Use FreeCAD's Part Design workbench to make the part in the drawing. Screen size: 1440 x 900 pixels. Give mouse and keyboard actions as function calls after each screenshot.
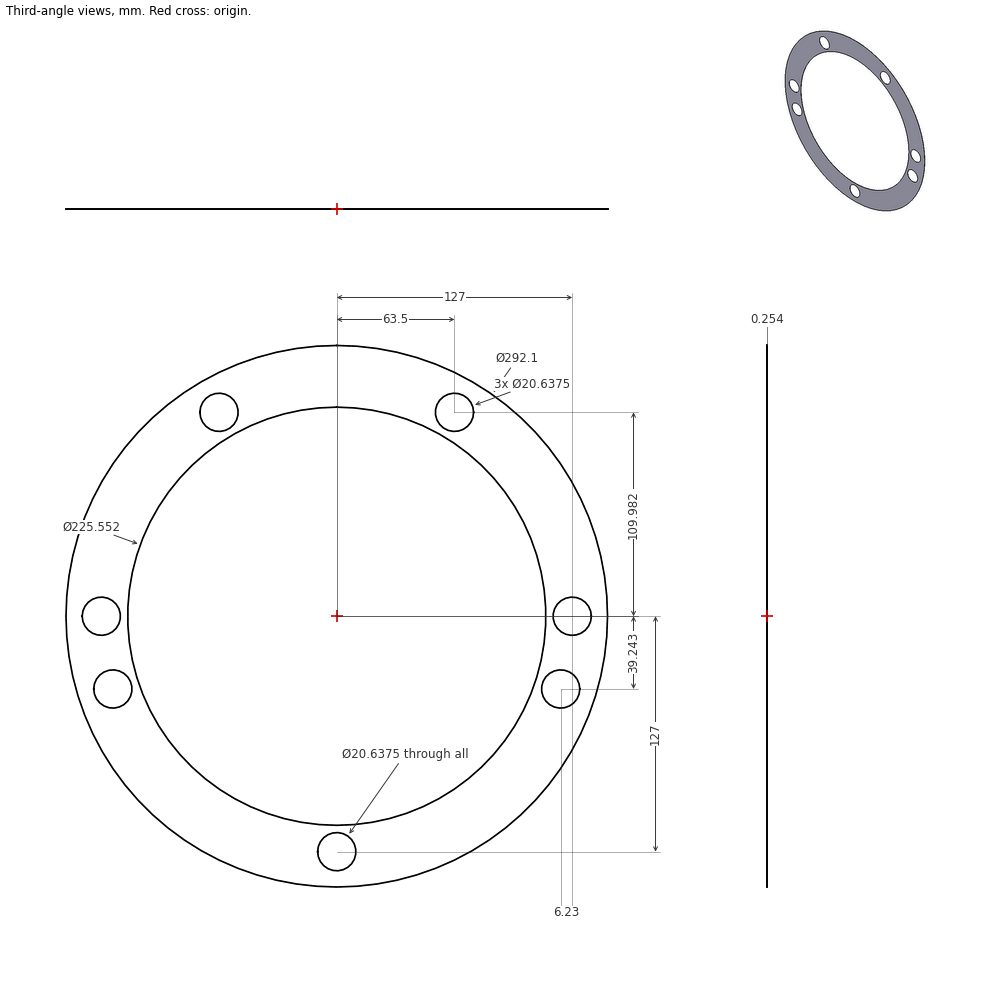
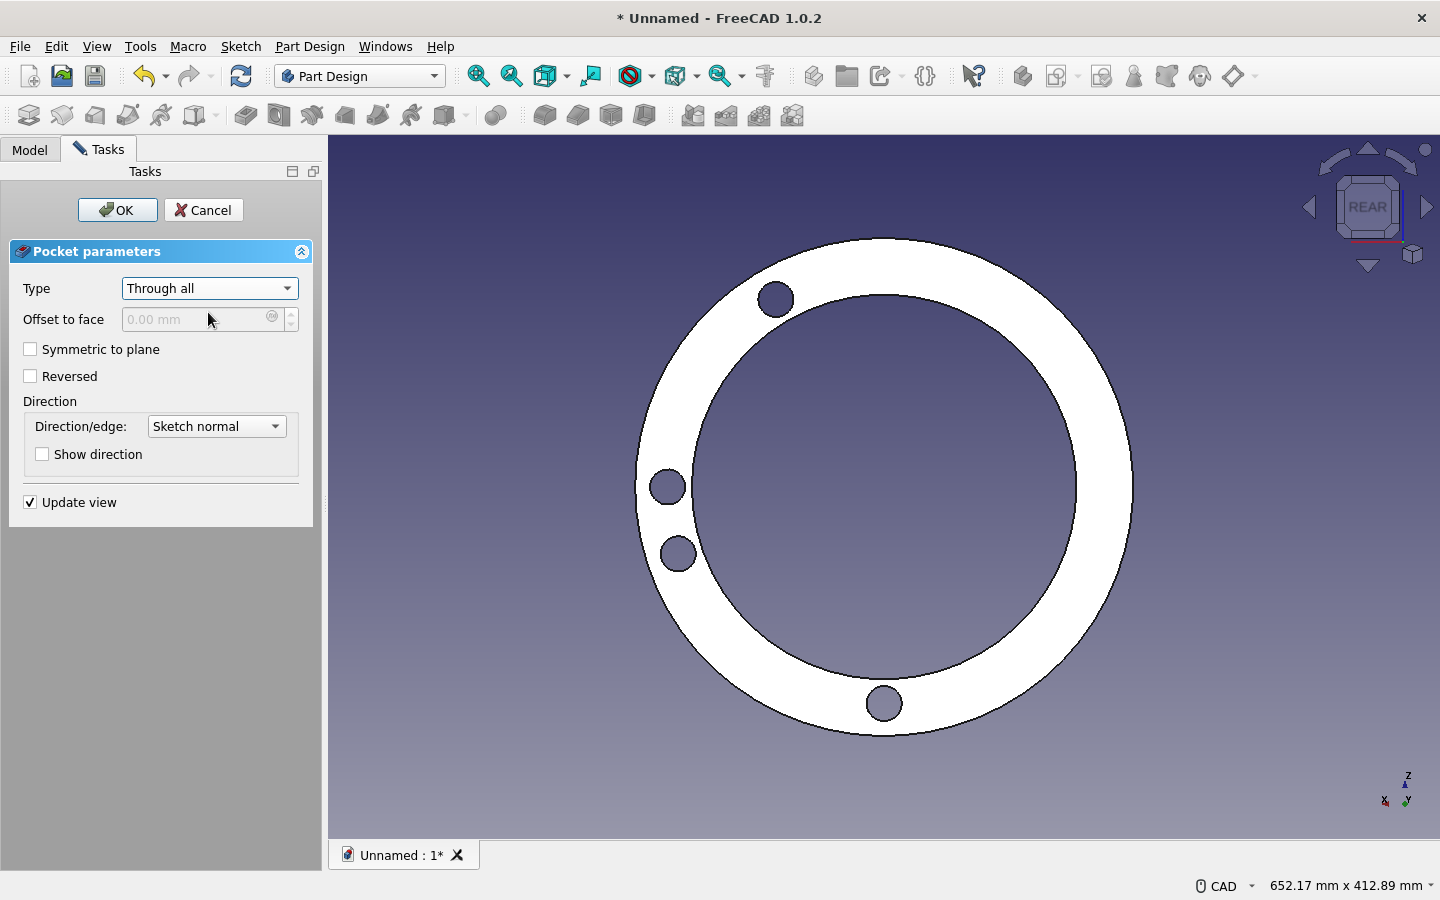
click(118, 210)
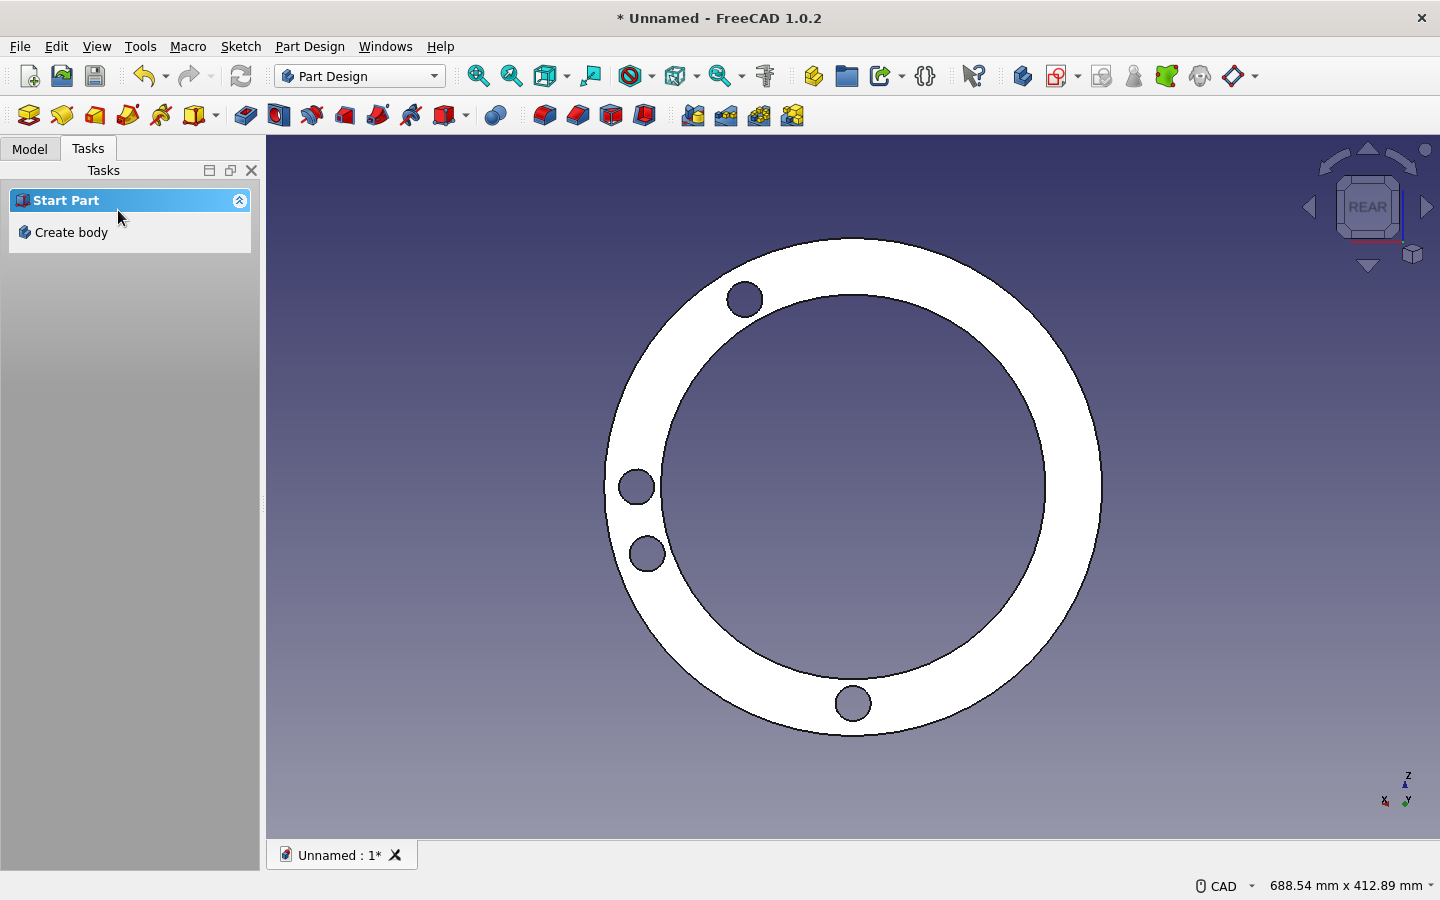
click(30, 148)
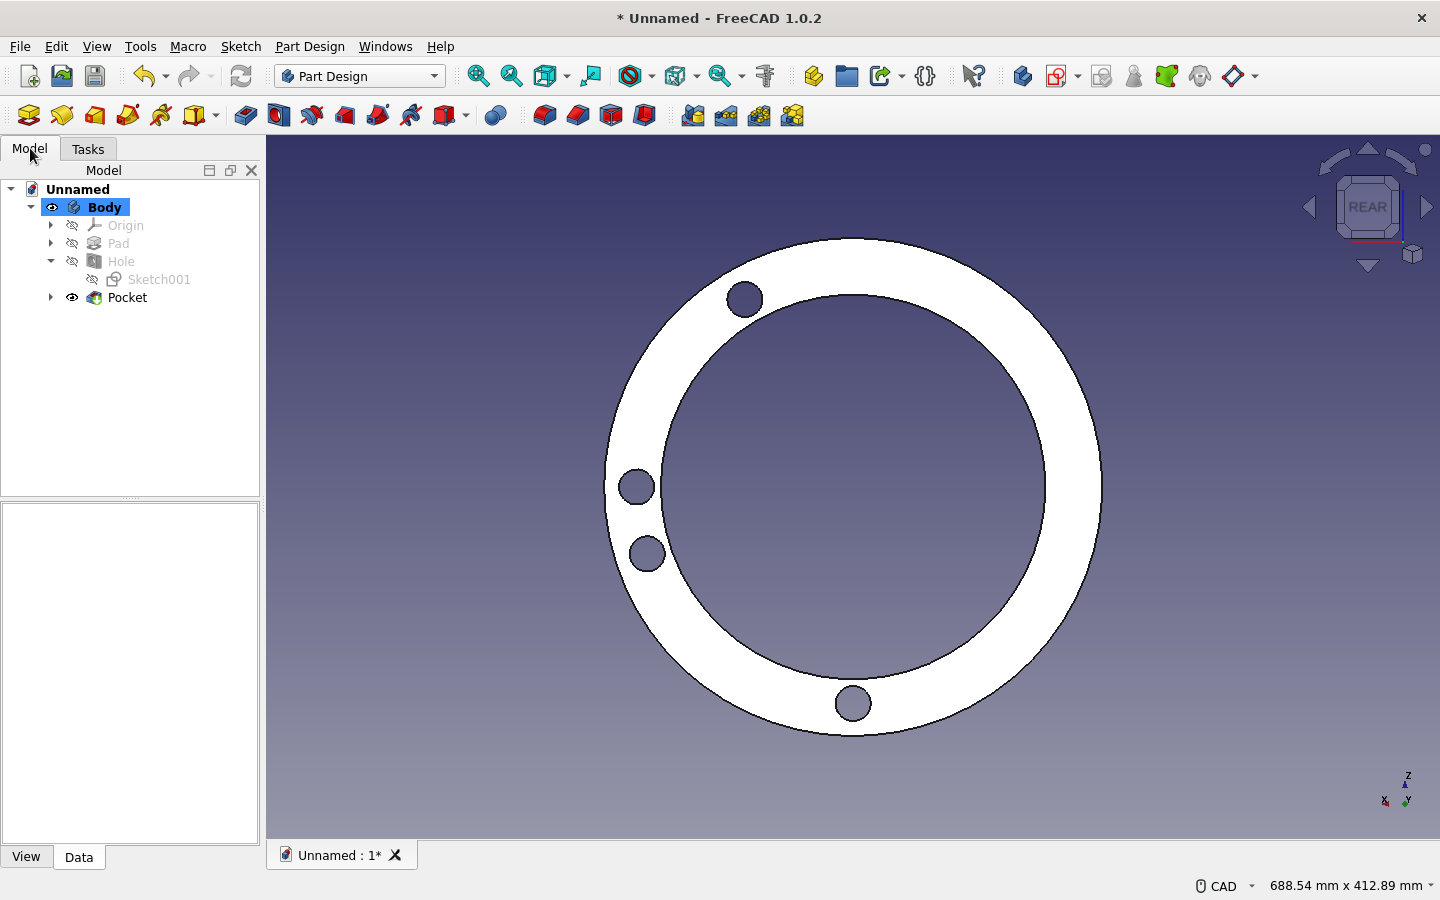
click(117, 297)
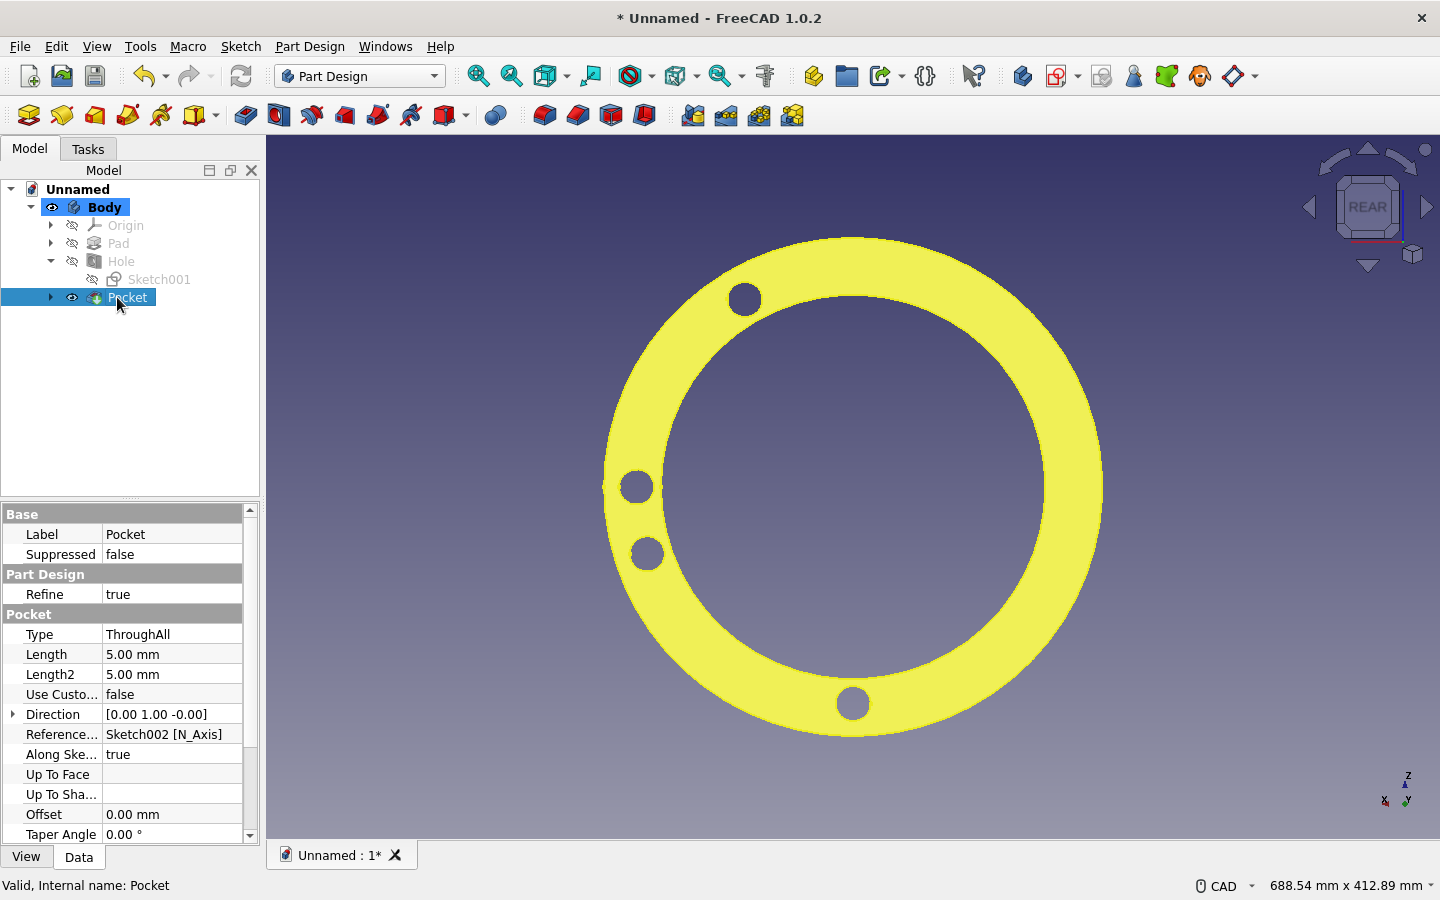
click(693, 116)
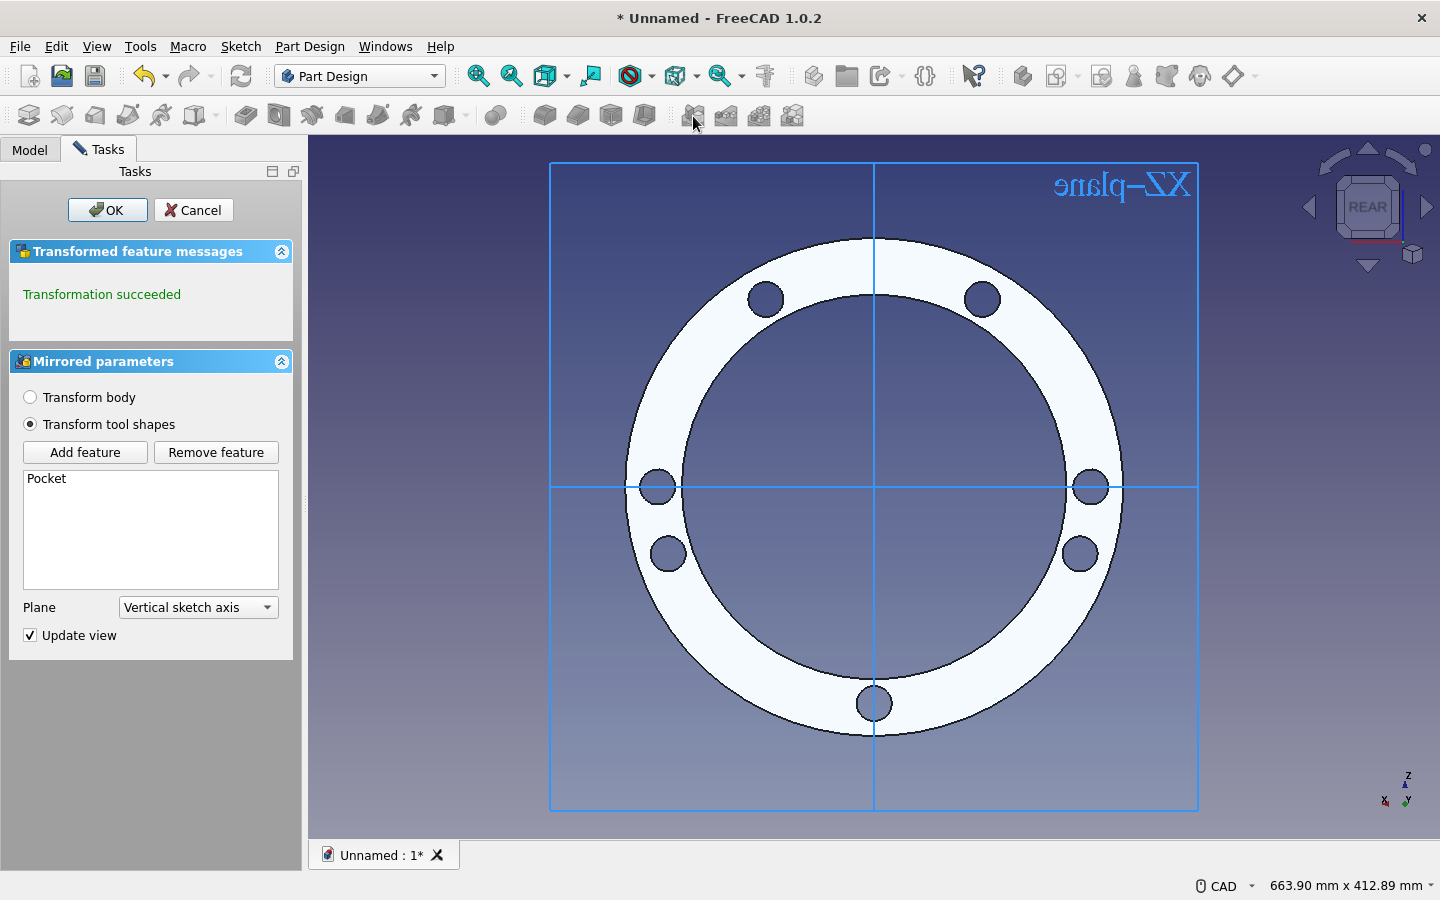
click(199, 608)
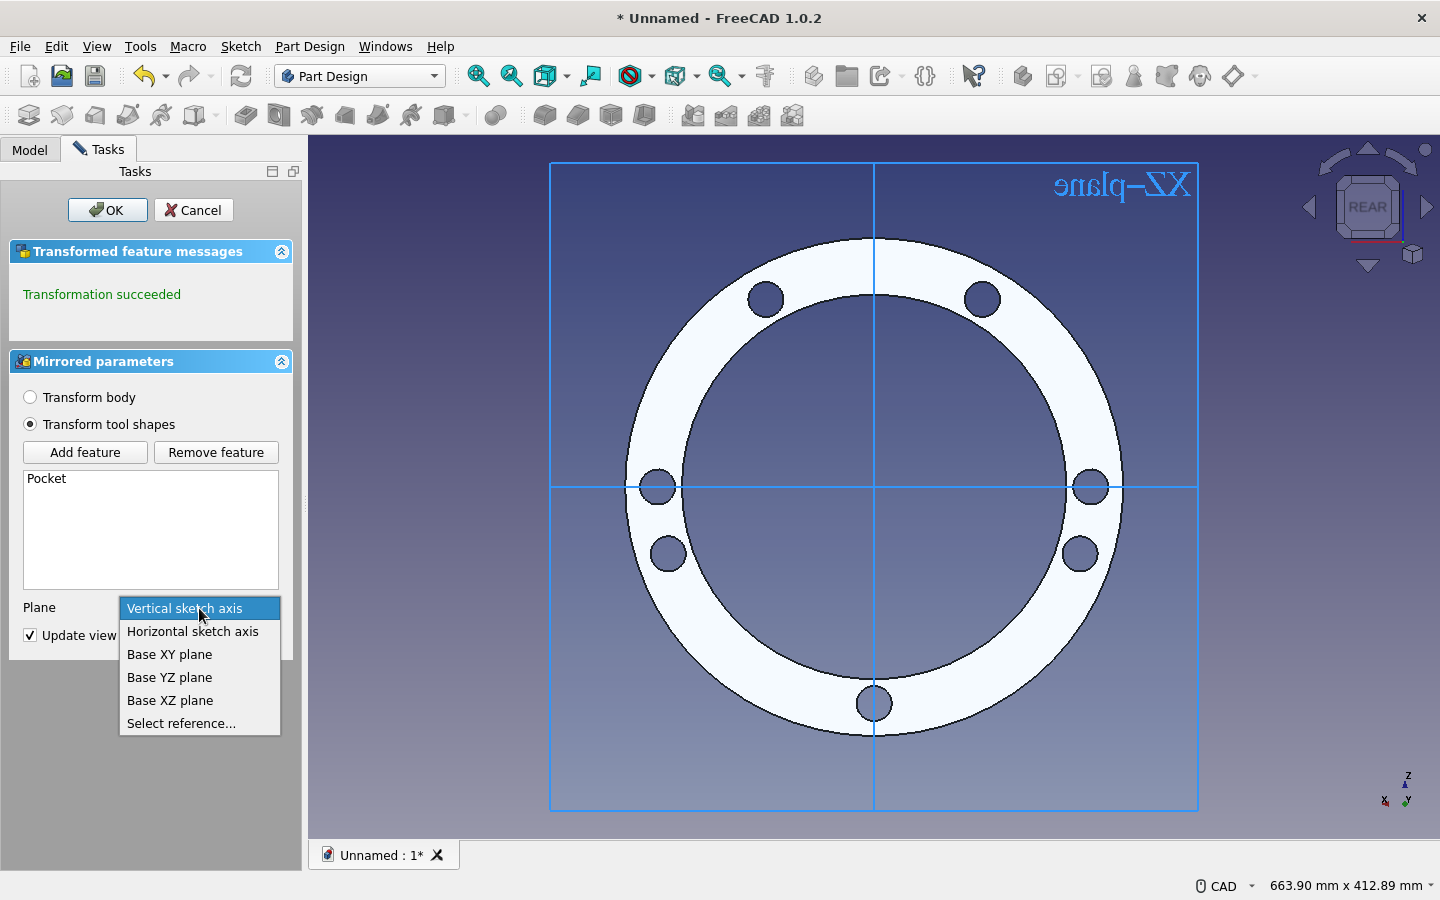
click(198, 678)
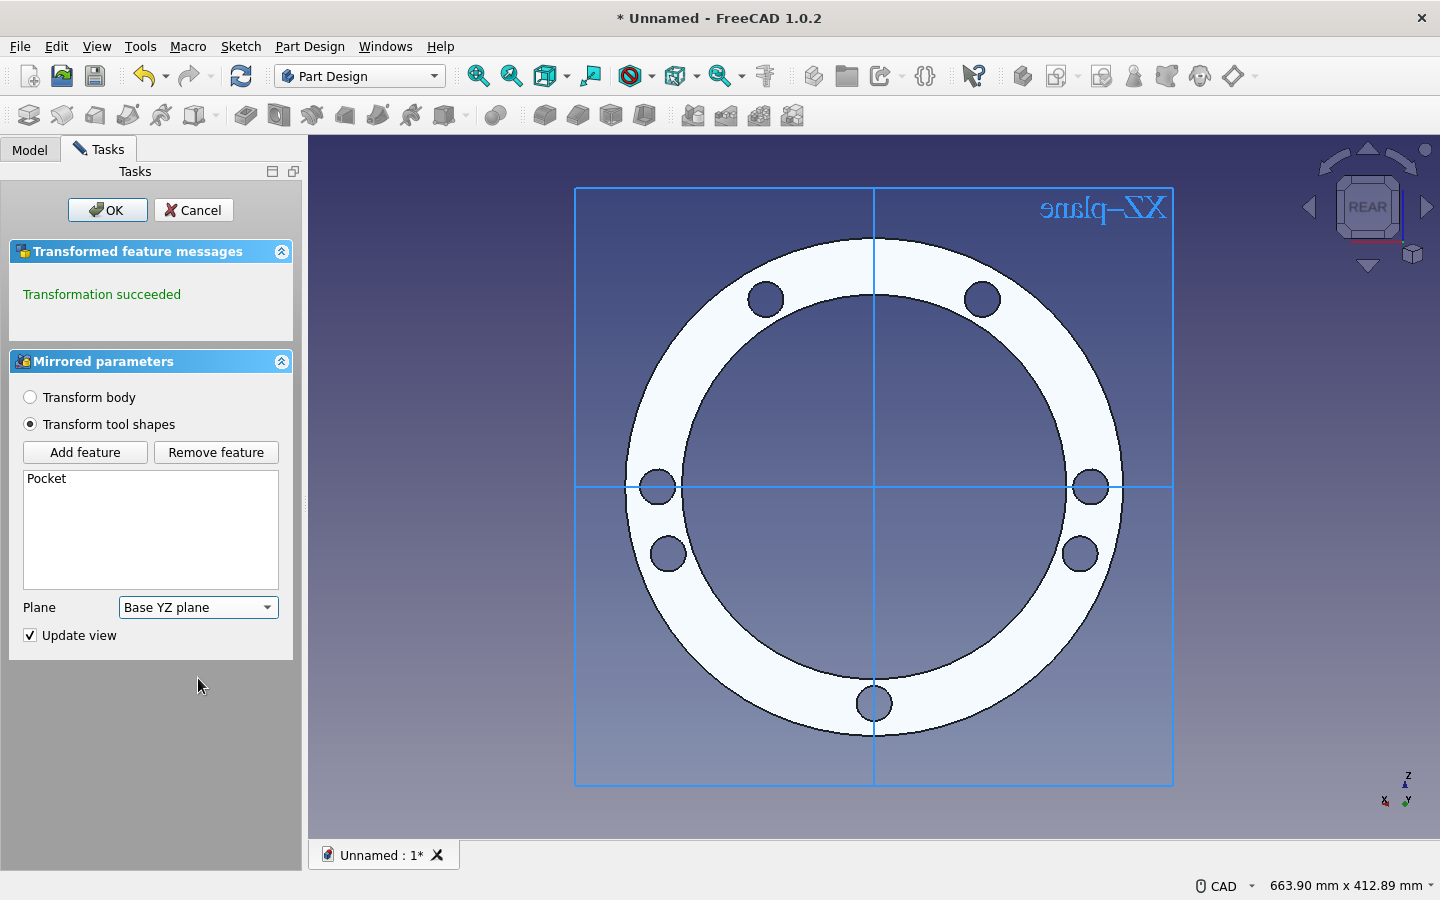
click(108, 210)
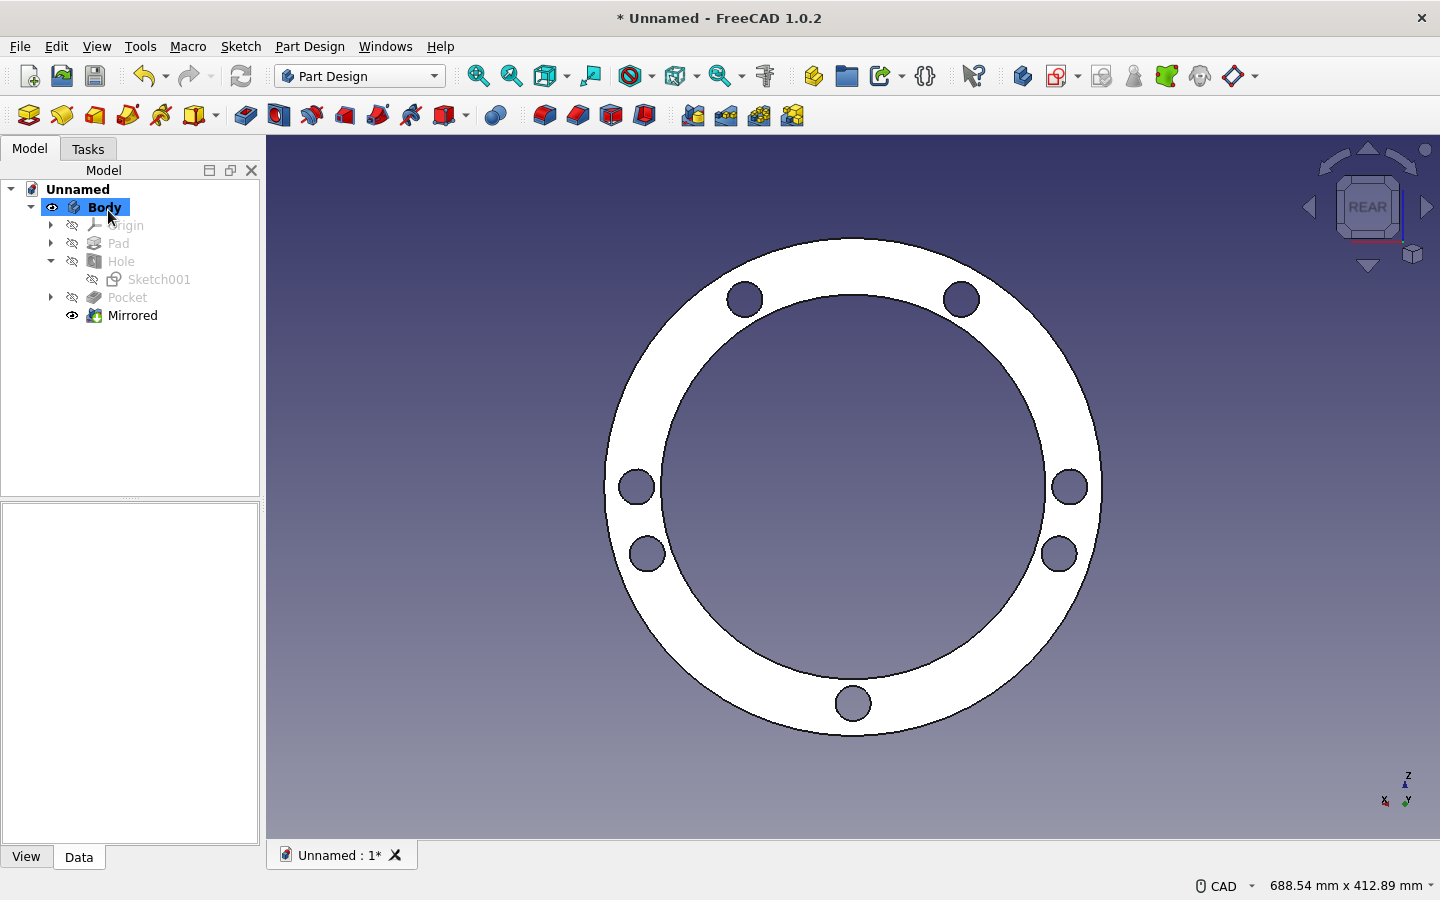
key(0)